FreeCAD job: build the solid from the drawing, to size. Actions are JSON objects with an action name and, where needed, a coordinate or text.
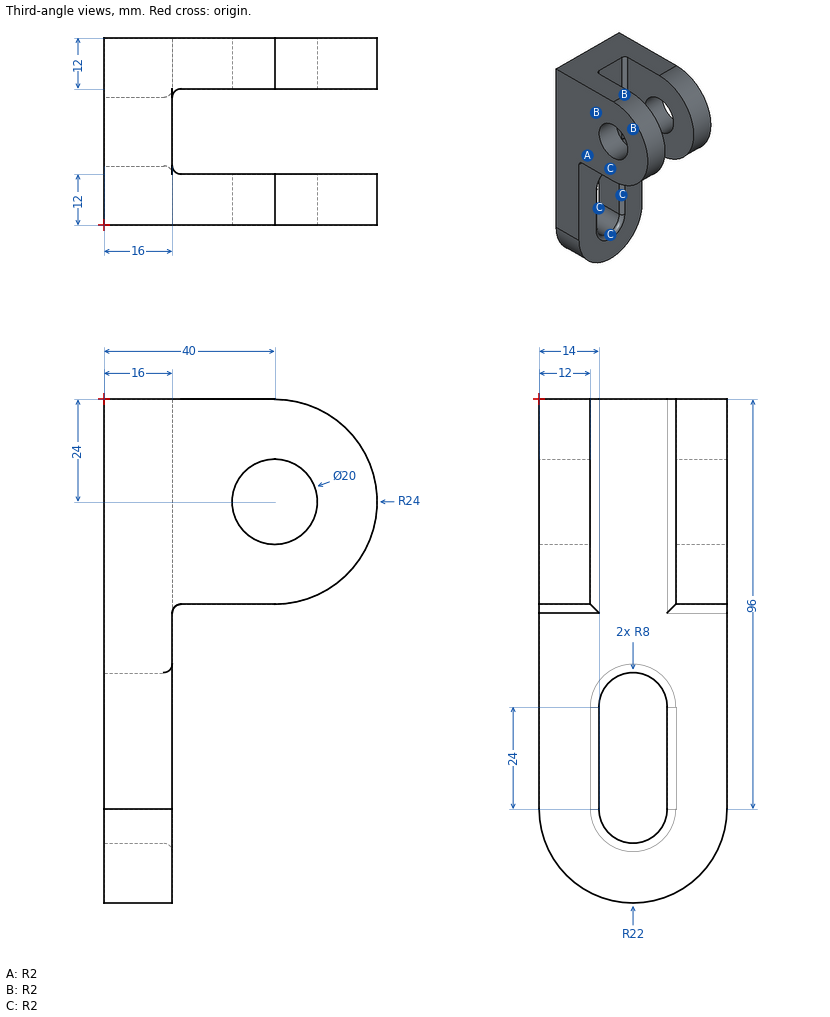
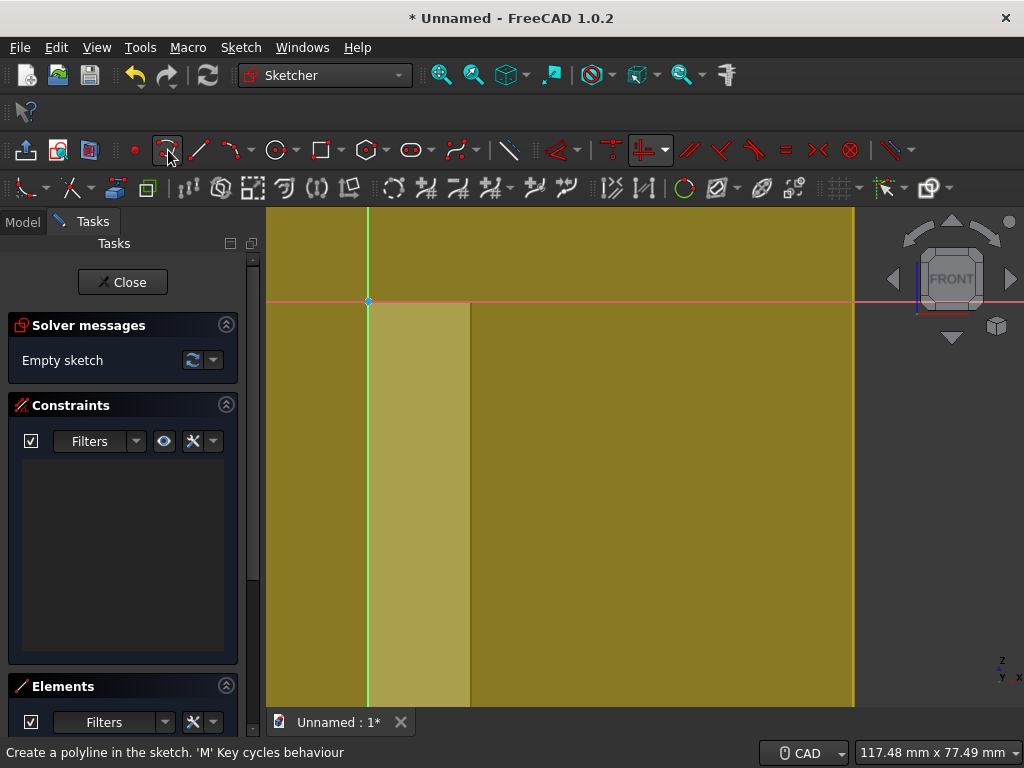
{"action": "left_click", "coordinate": [626, 612]}
{"action": "left_click", "coordinate": [368, 612]}
{"action": "left_click", "coordinate": [368, 302]}
{"action": "left_click", "coordinate": [626, 311]}
{"action": "right_click", "coordinate": [626, 311]}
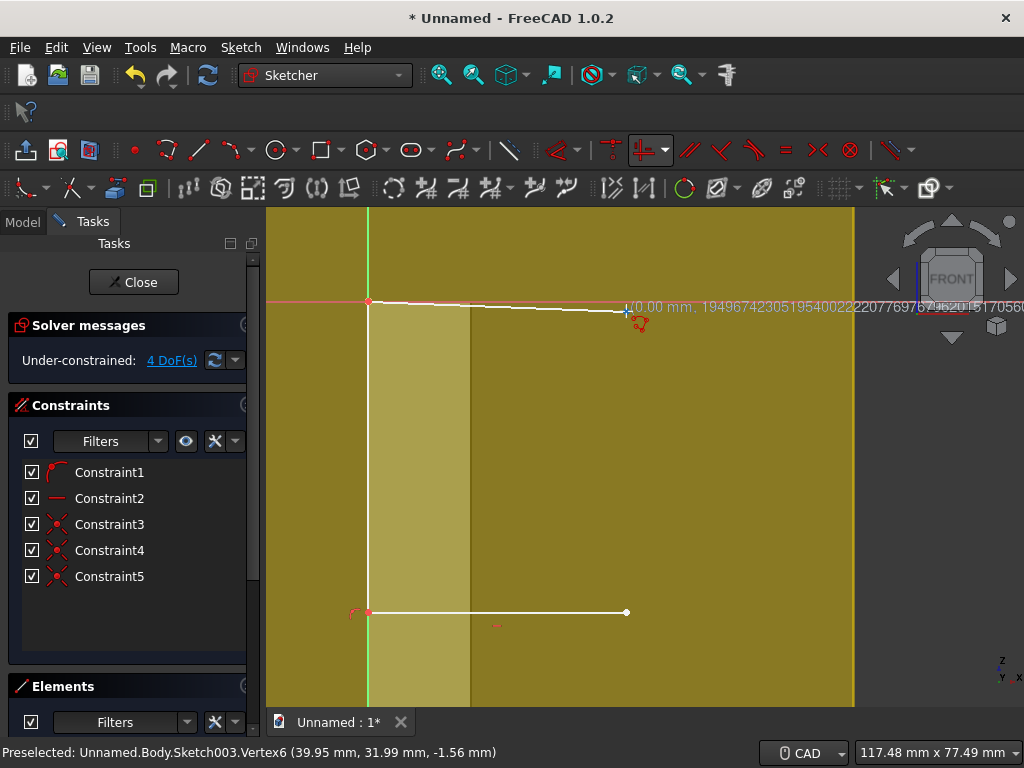
{"action": "left_click", "coordinate": [232, 150]}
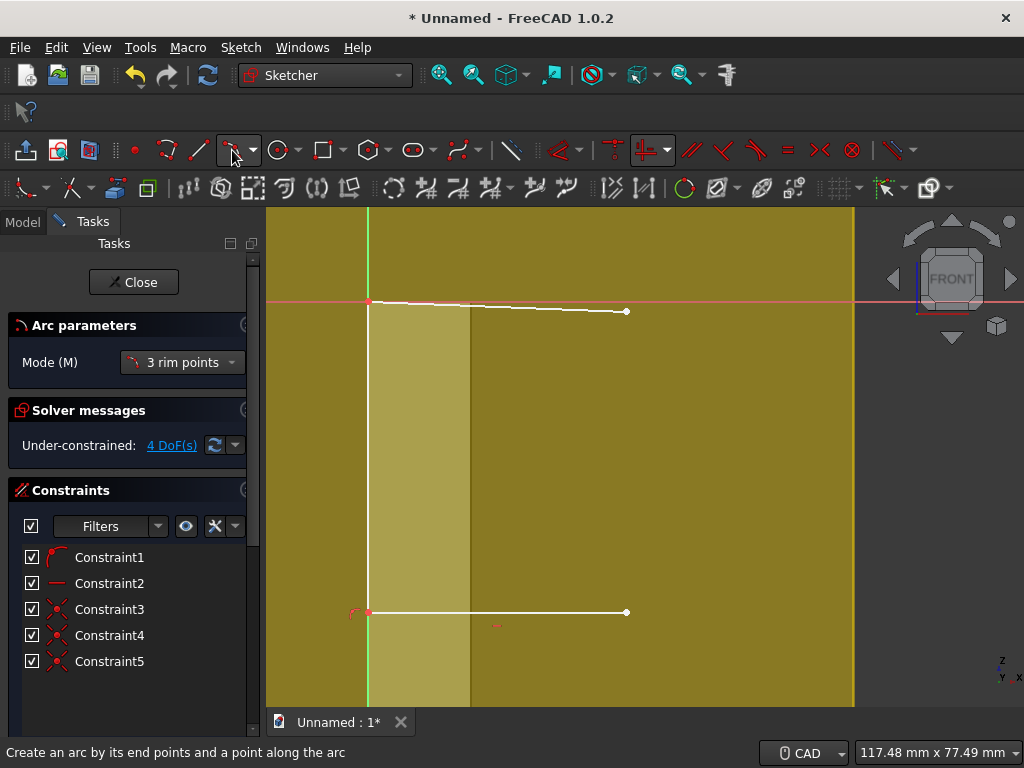
{"action": "left_click", "coordinate": [626, 312]}
{"action": "left_click", "coordinate": [626, 613]}
{"action": "left_click", "coordinate": [781, 457]}
{"action": "key", "text": "Escape"}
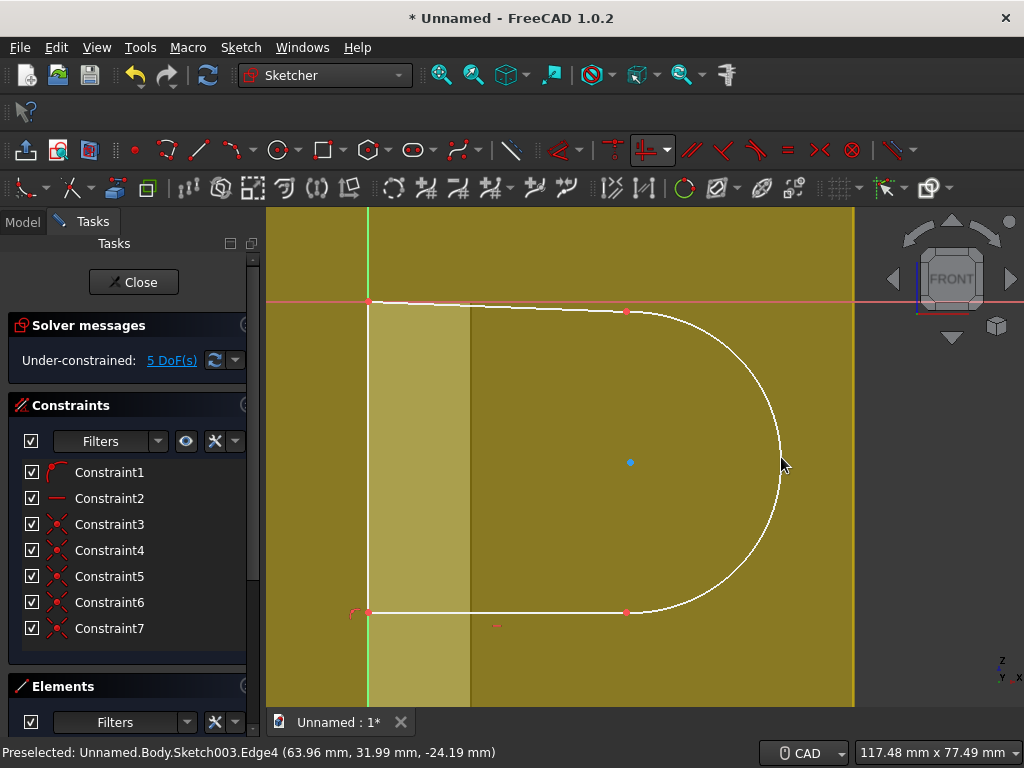
{"action": "left_click", "coordinate": [549, 613]}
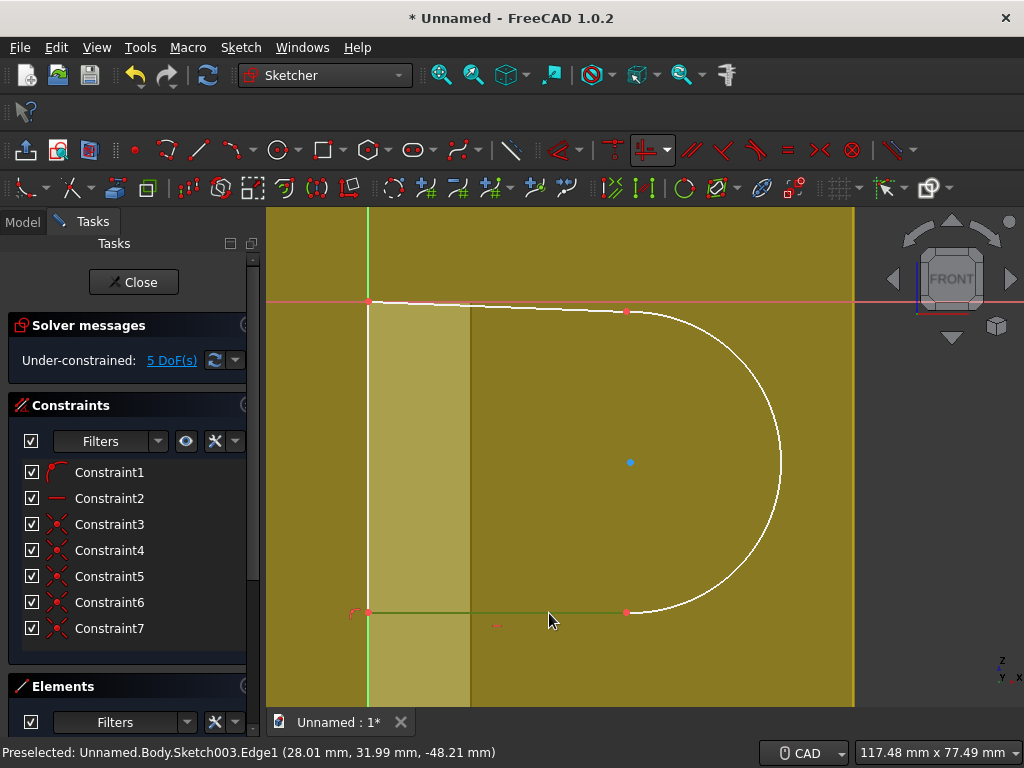
{"action": "left_click", "coordinate": [751, 552]}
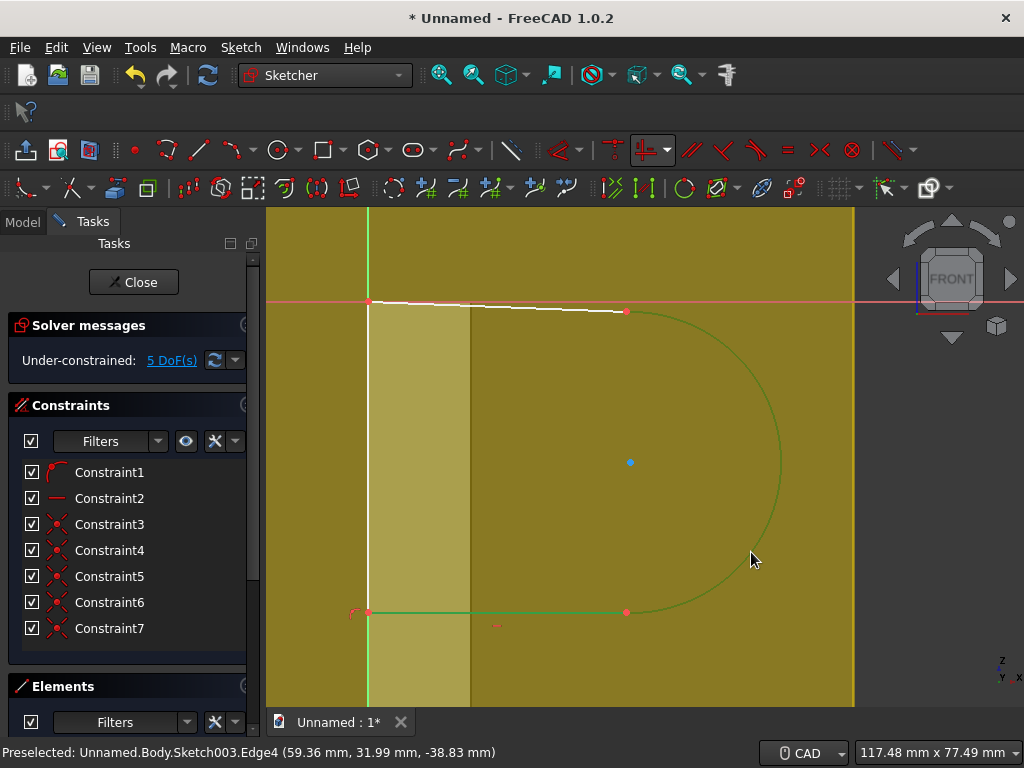
{"action": "left_click", "coordinate": [756, 150]}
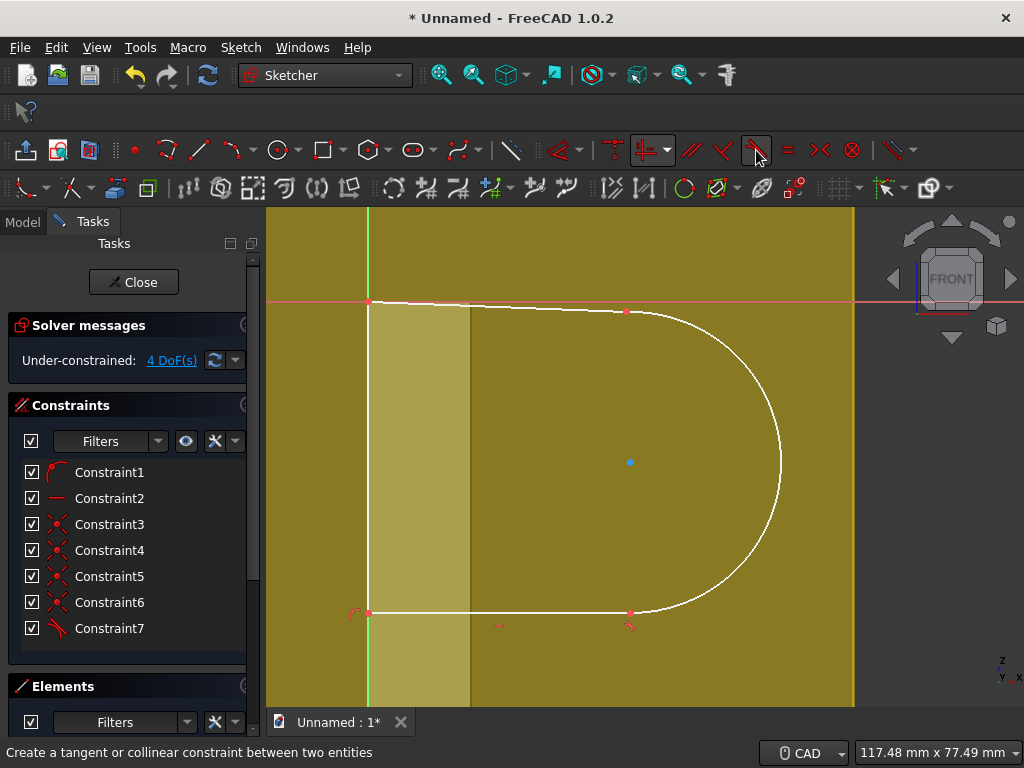
{"action": "left_click", "coordinate": [446, 305]}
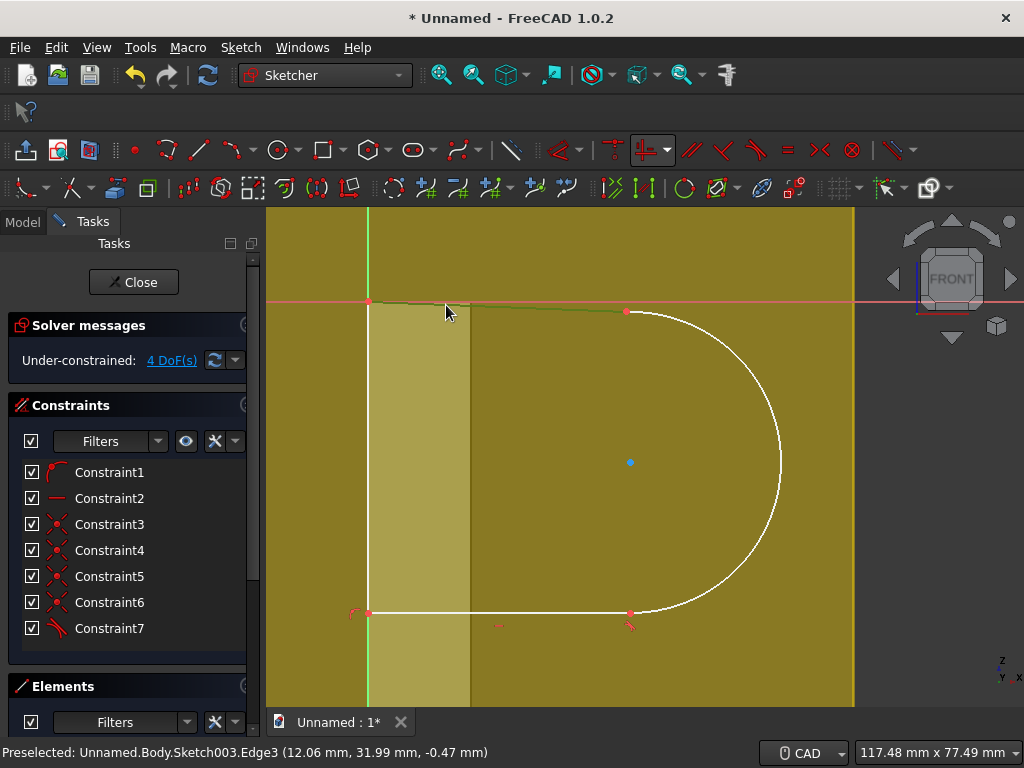
{"action": "left_click", "coordinate": [753, 550]}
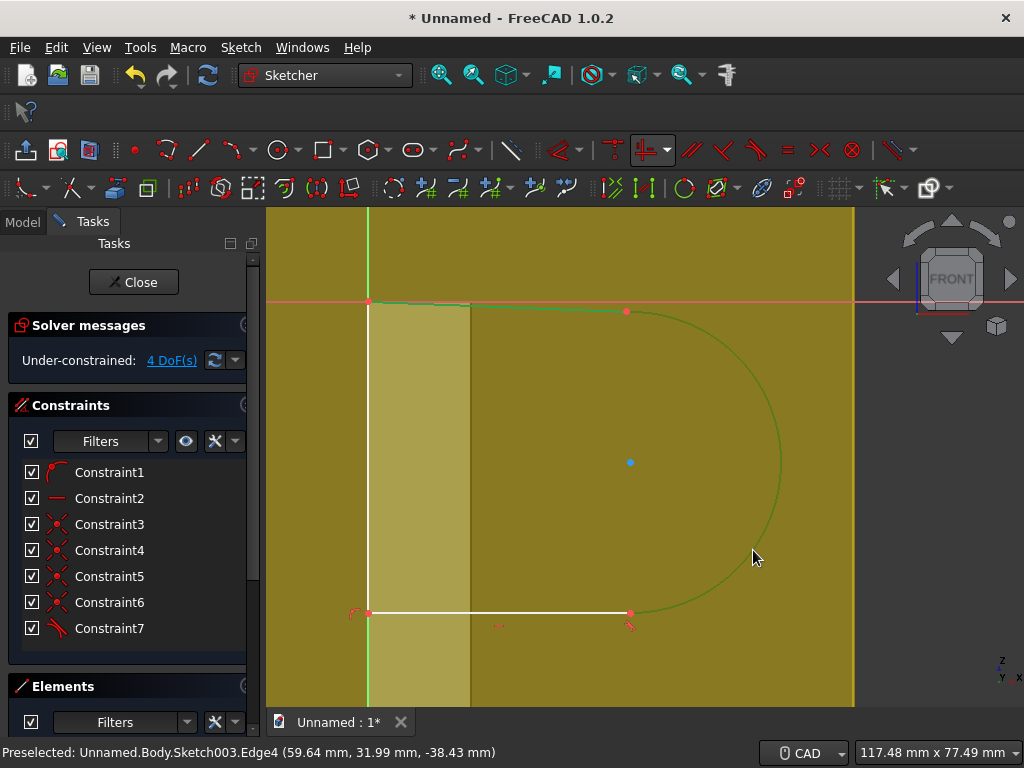
{"action": "left_click", "coordinate": [756, 150]}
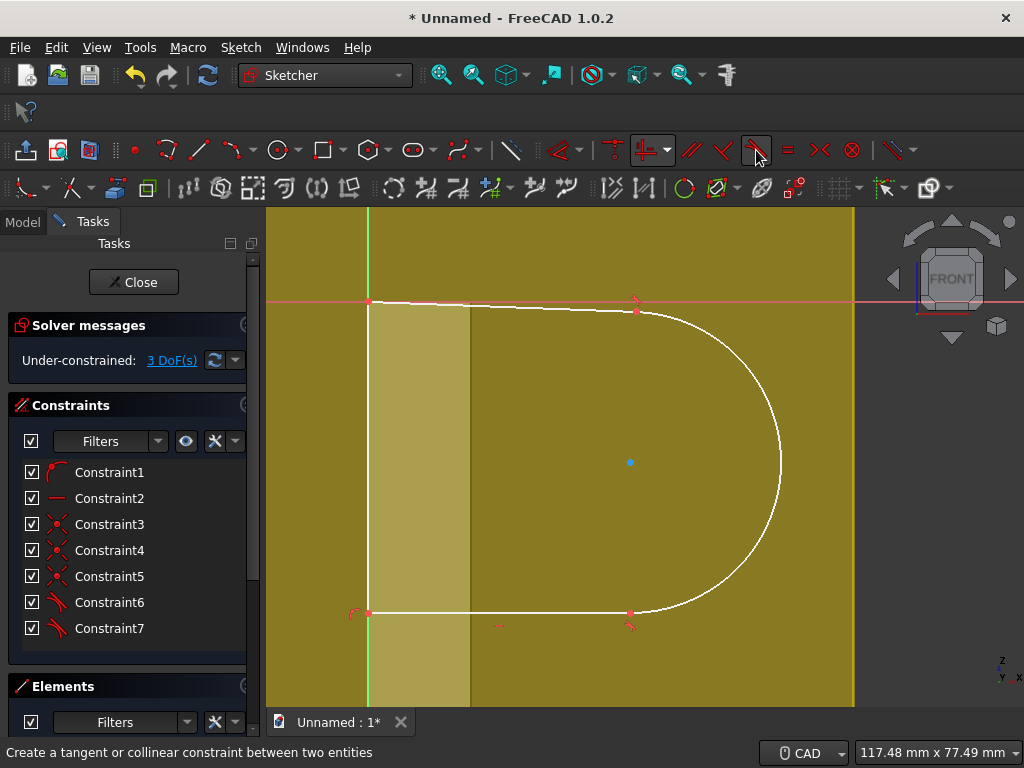
{"action": "left_click", "coordinate": [449, 305]}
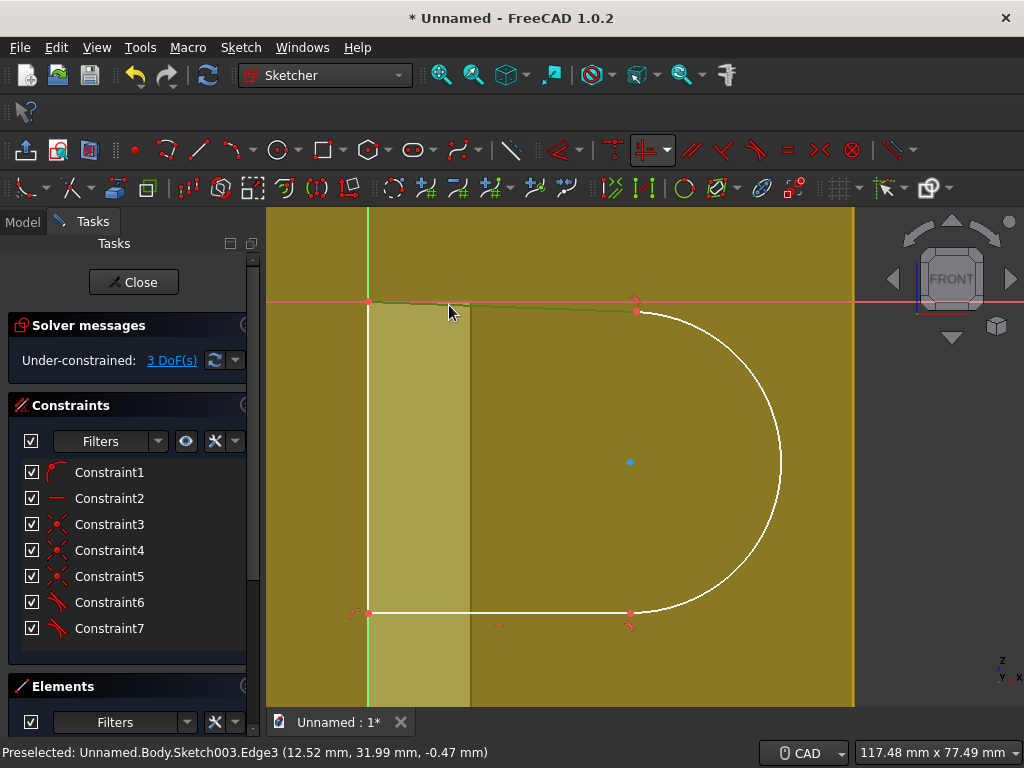
{"action": "key", "text": "h"}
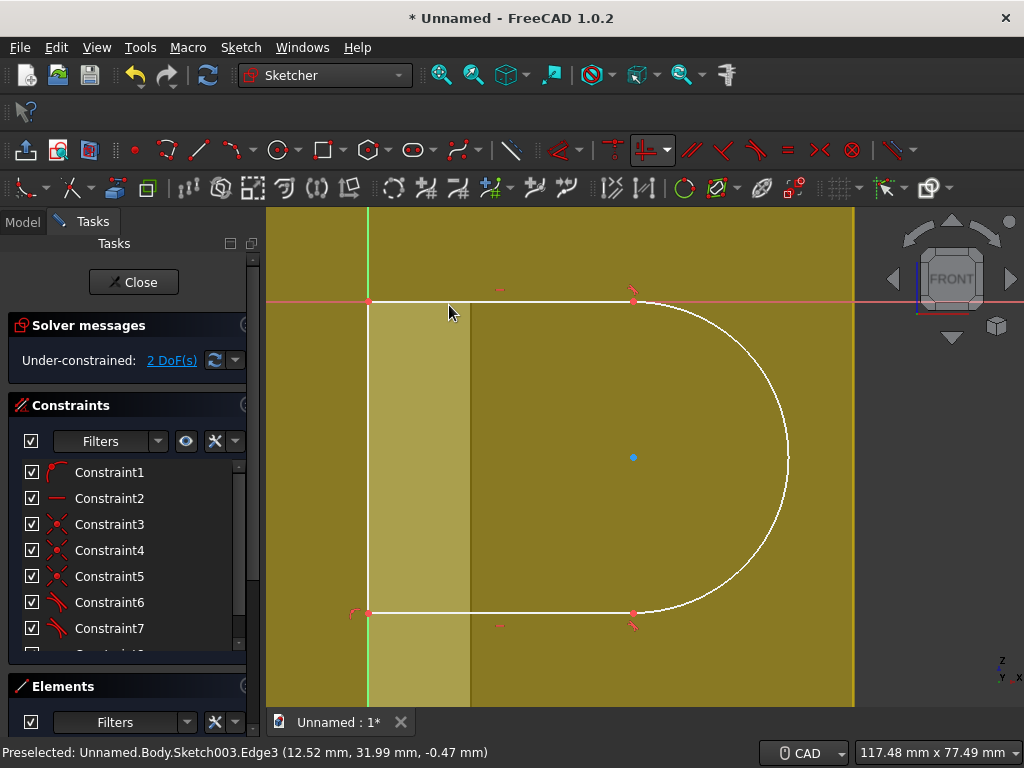
{"action": "key", "text": "d"}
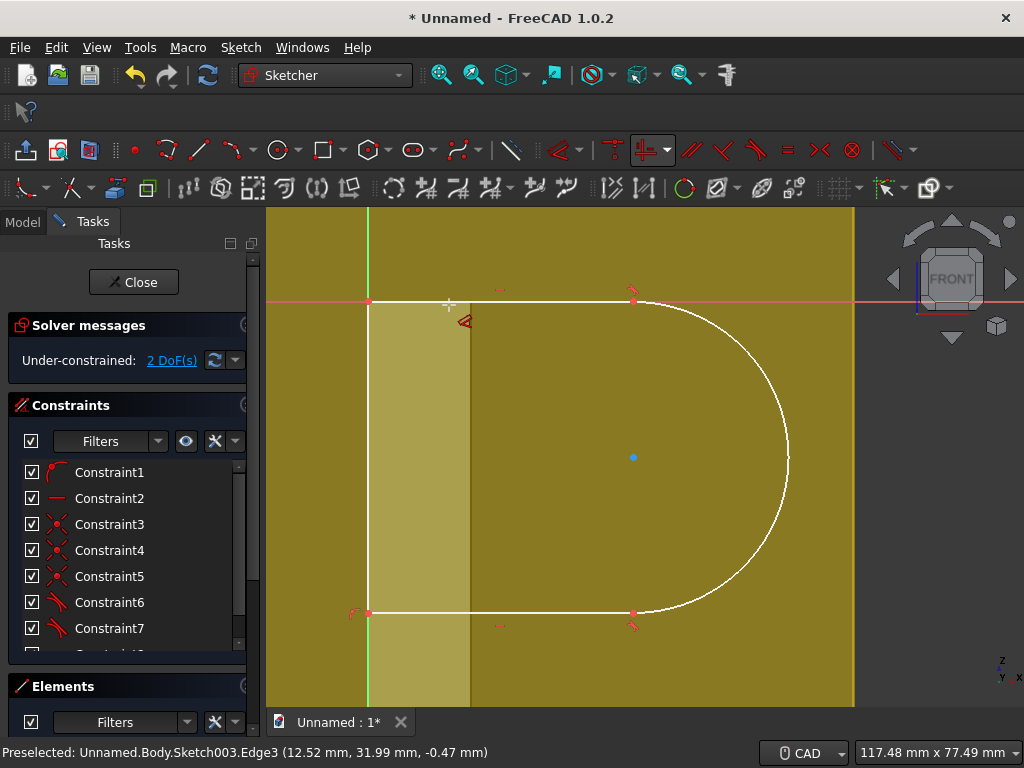
{"action": "left_click", "coordinate": [759, 549]}
{"action": "left_click", "coordinate": [785, 568]}